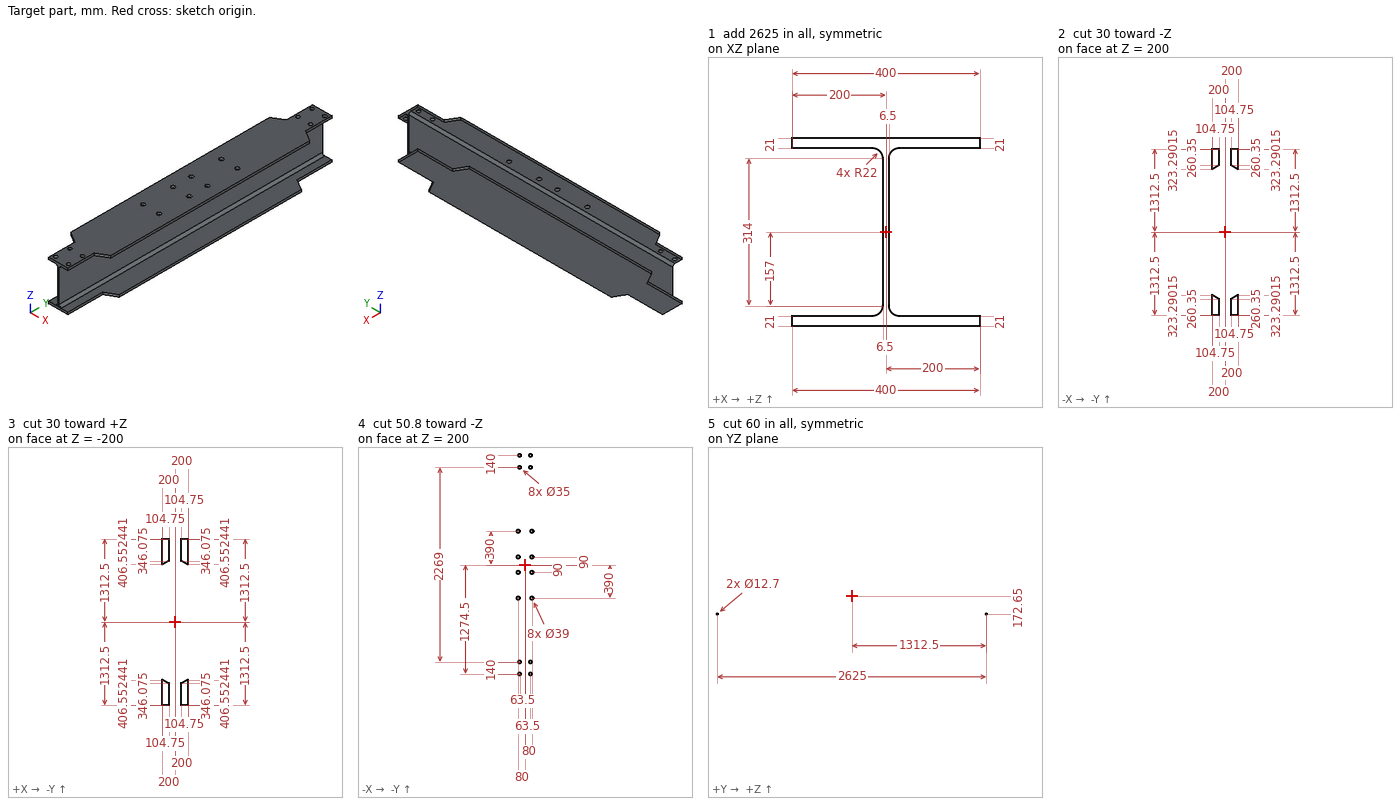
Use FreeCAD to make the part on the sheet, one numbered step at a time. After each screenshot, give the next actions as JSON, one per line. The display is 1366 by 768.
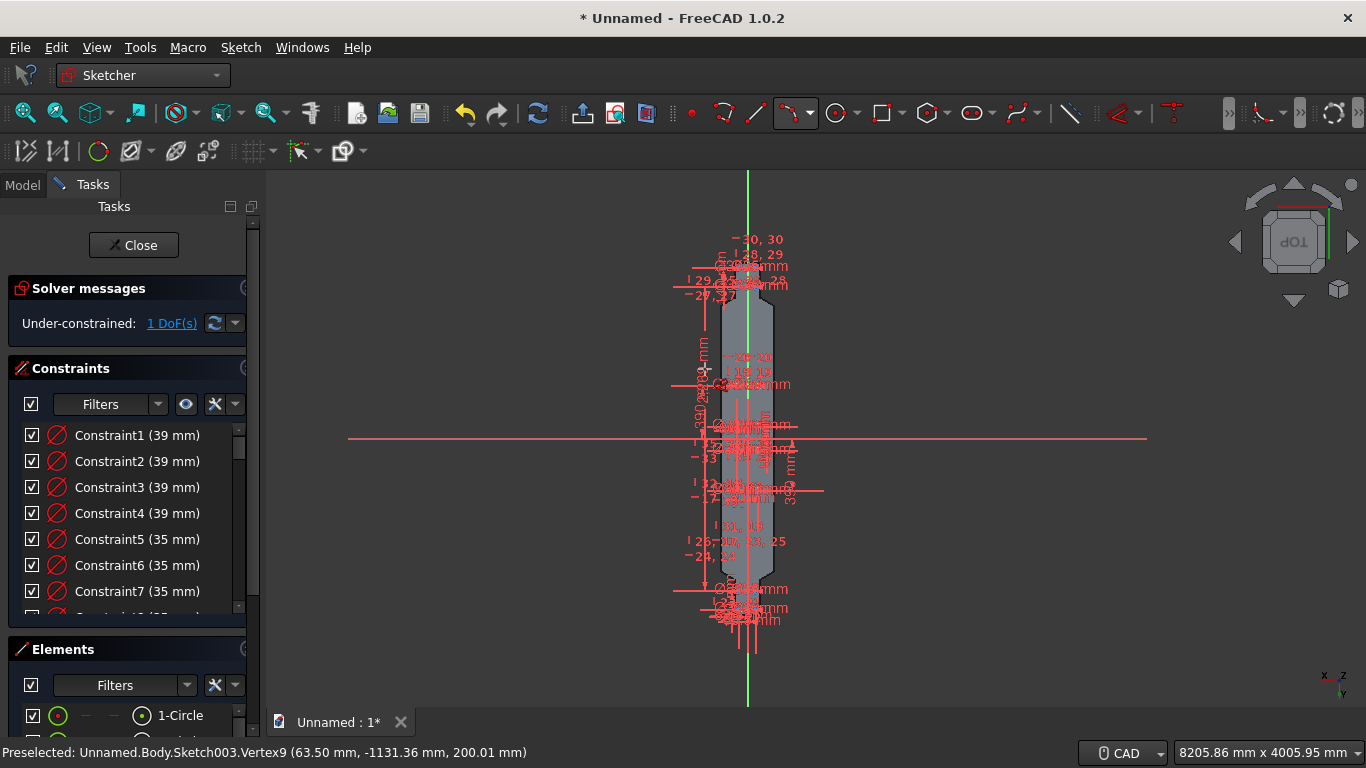
{"action": "left_click", "coordinate": [739, 610]}
{"action": "left_click", "coordinate": [705, 524]}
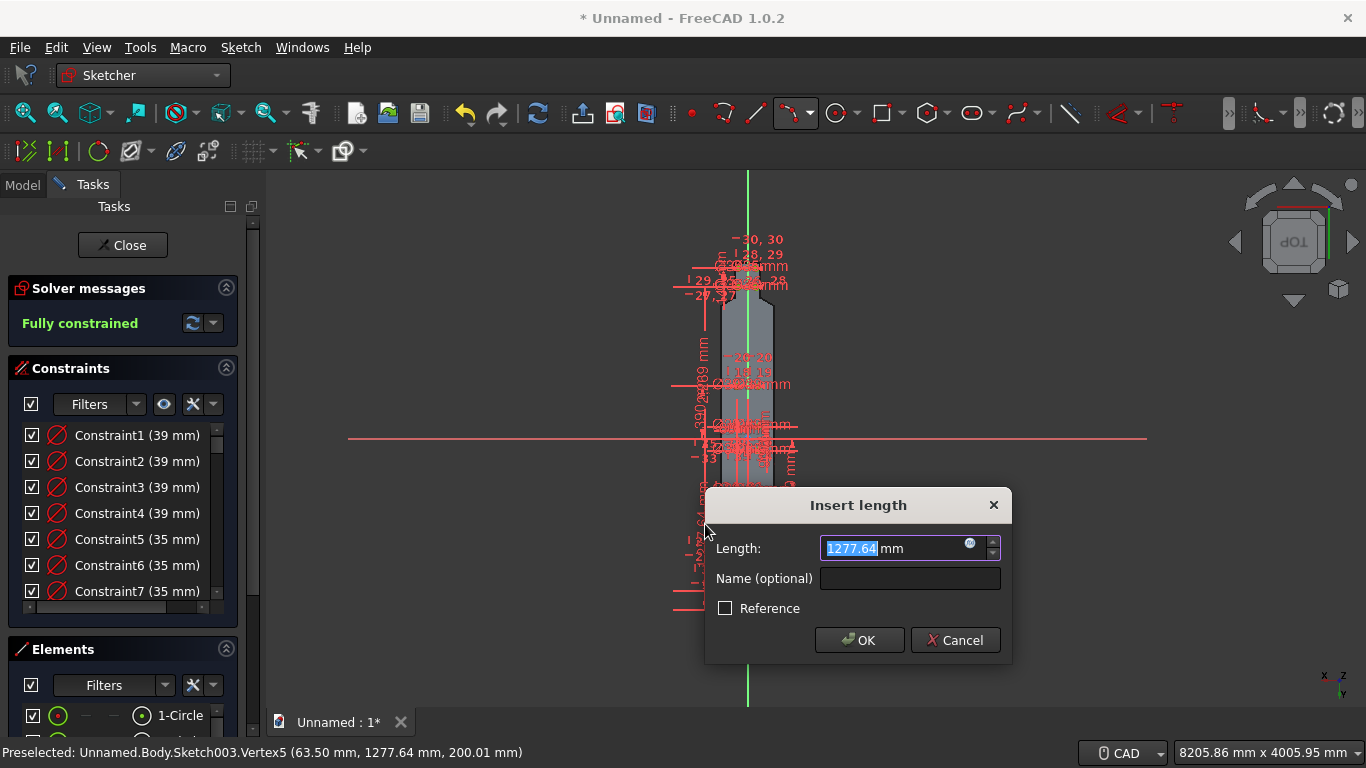
{"action": "type", "text": "1274.5"}
{"action": "key", "text": "Return"}
{"action": "key", "text": "Escape"}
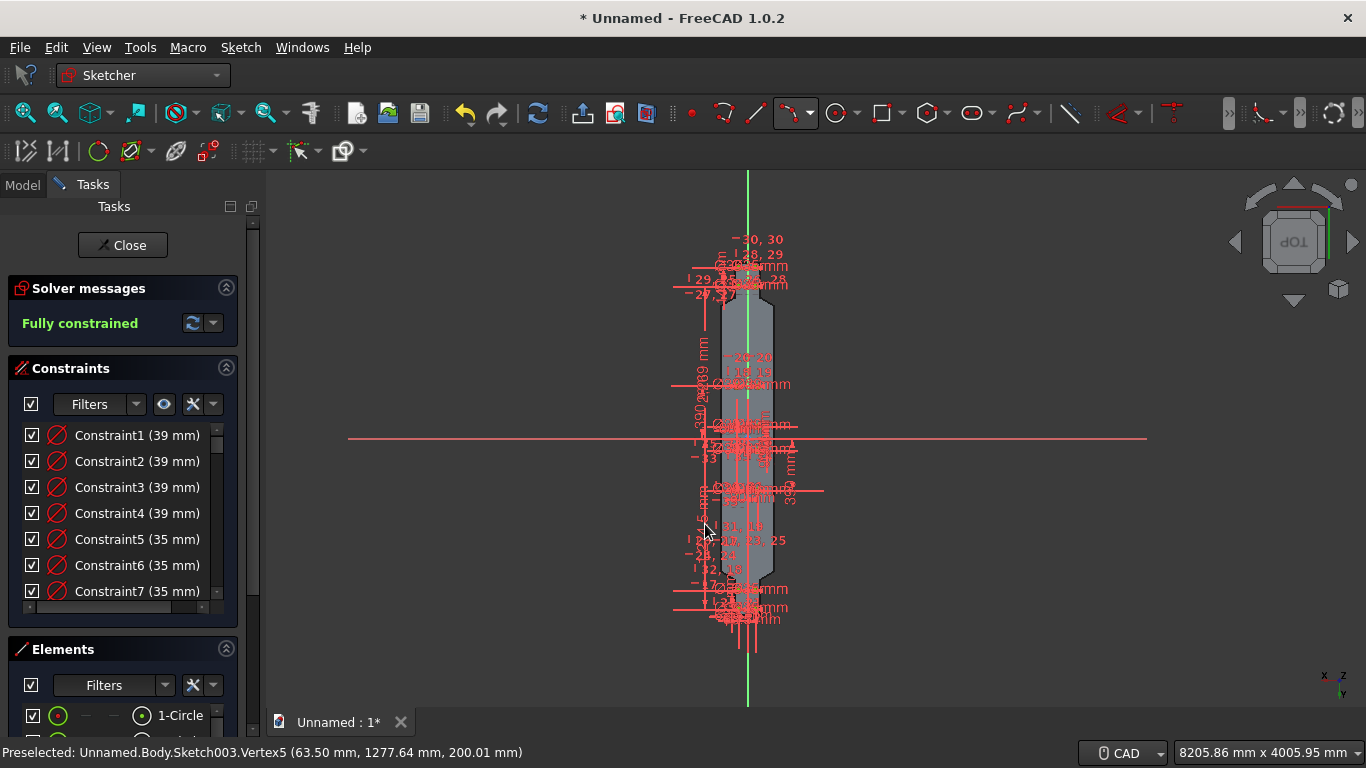
{"action": "left_click", "coordinate": [123, 245]}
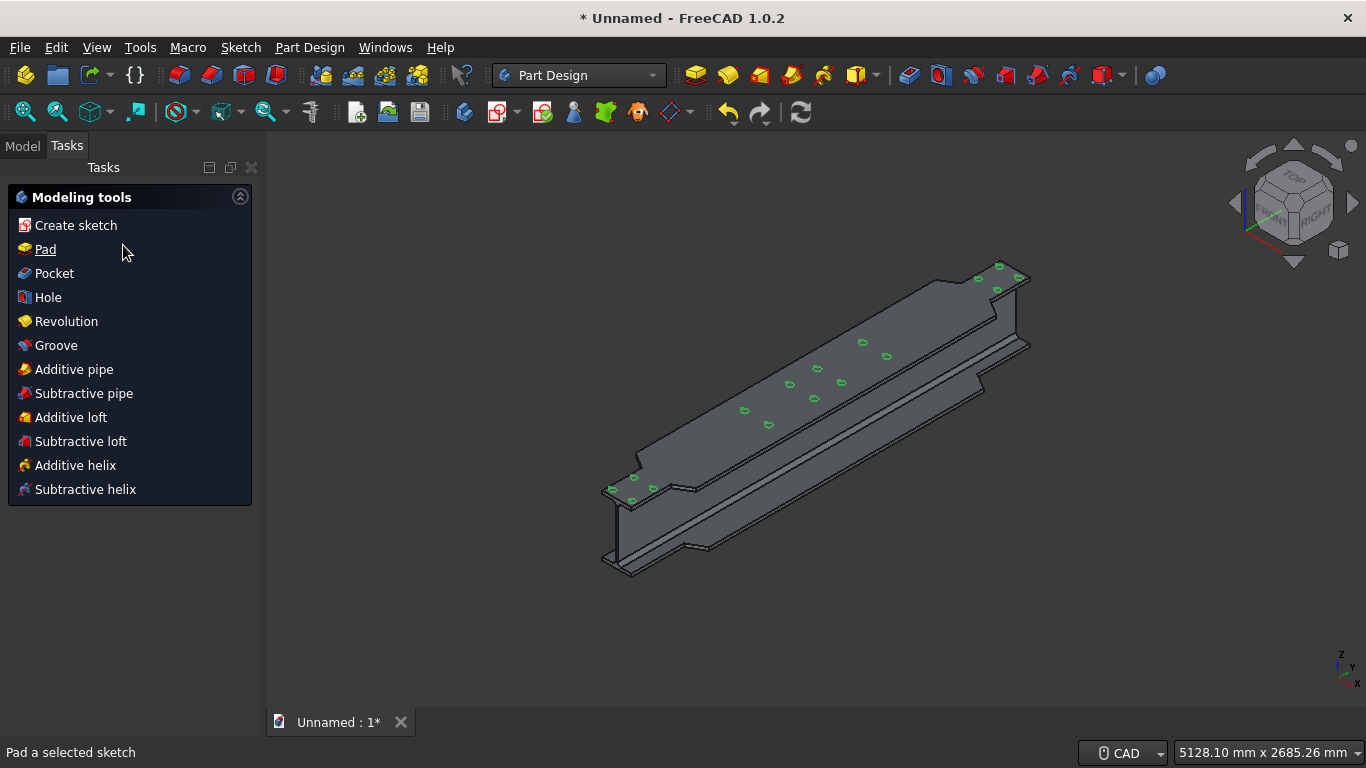
{"action": "left_click", "coordinate": [910, 76]}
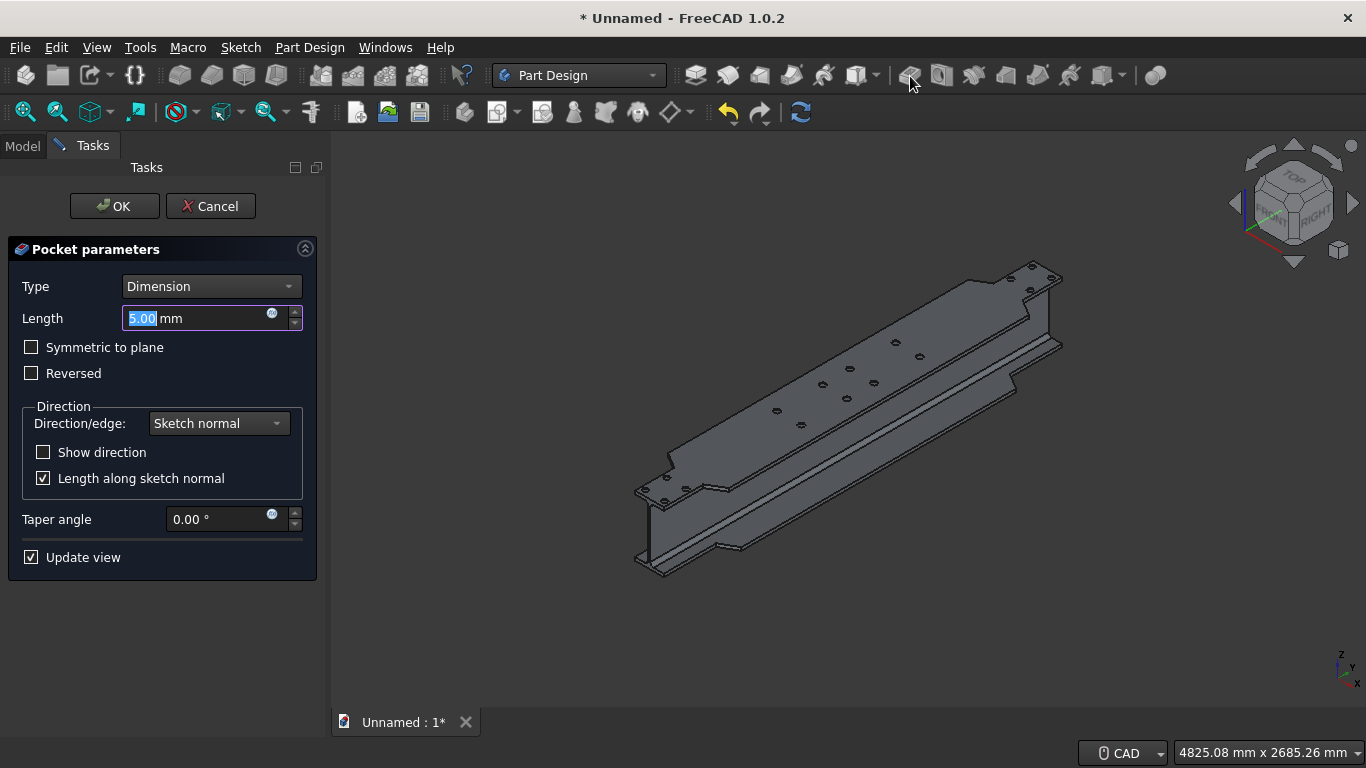
{"action": "type", "text": "50.8"}
{"action": "key", "text": "Tab"}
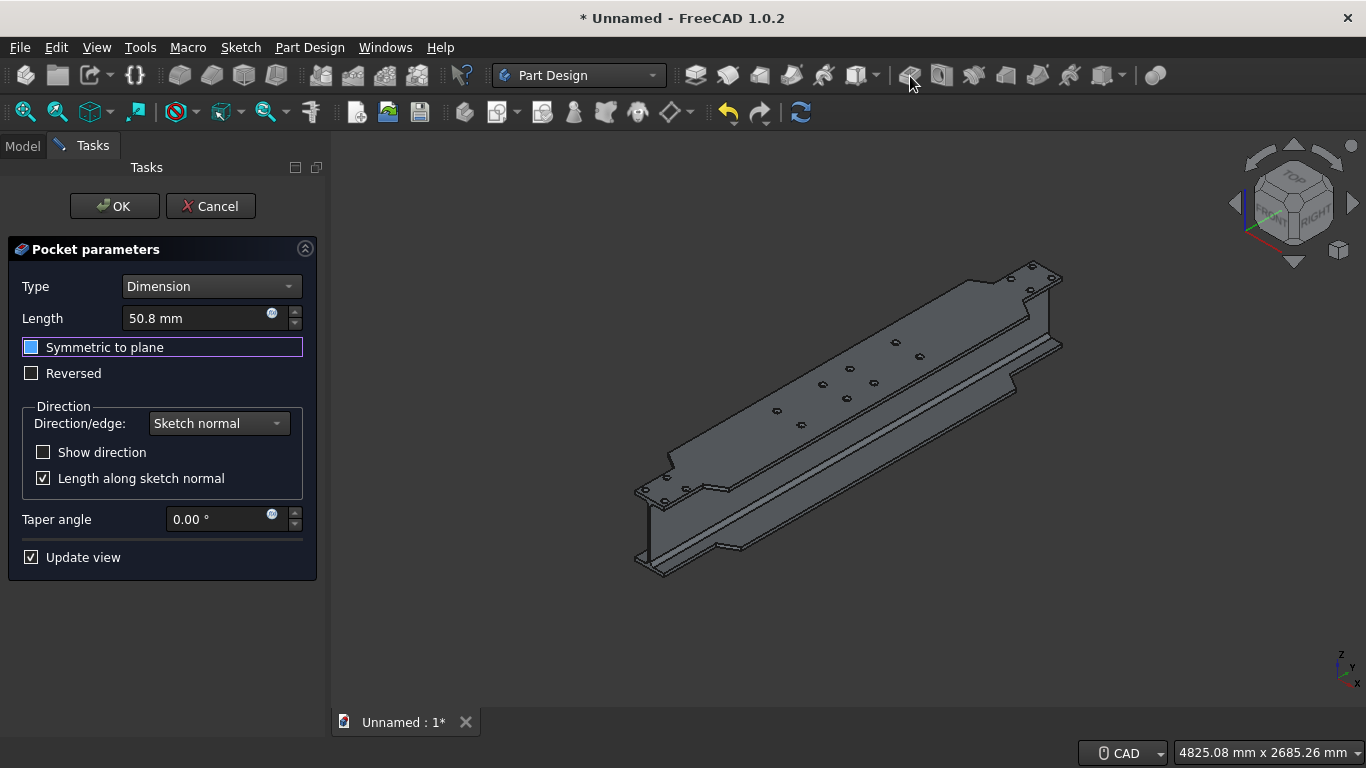
{"action": "left_click", "coordinate": [115, 206]}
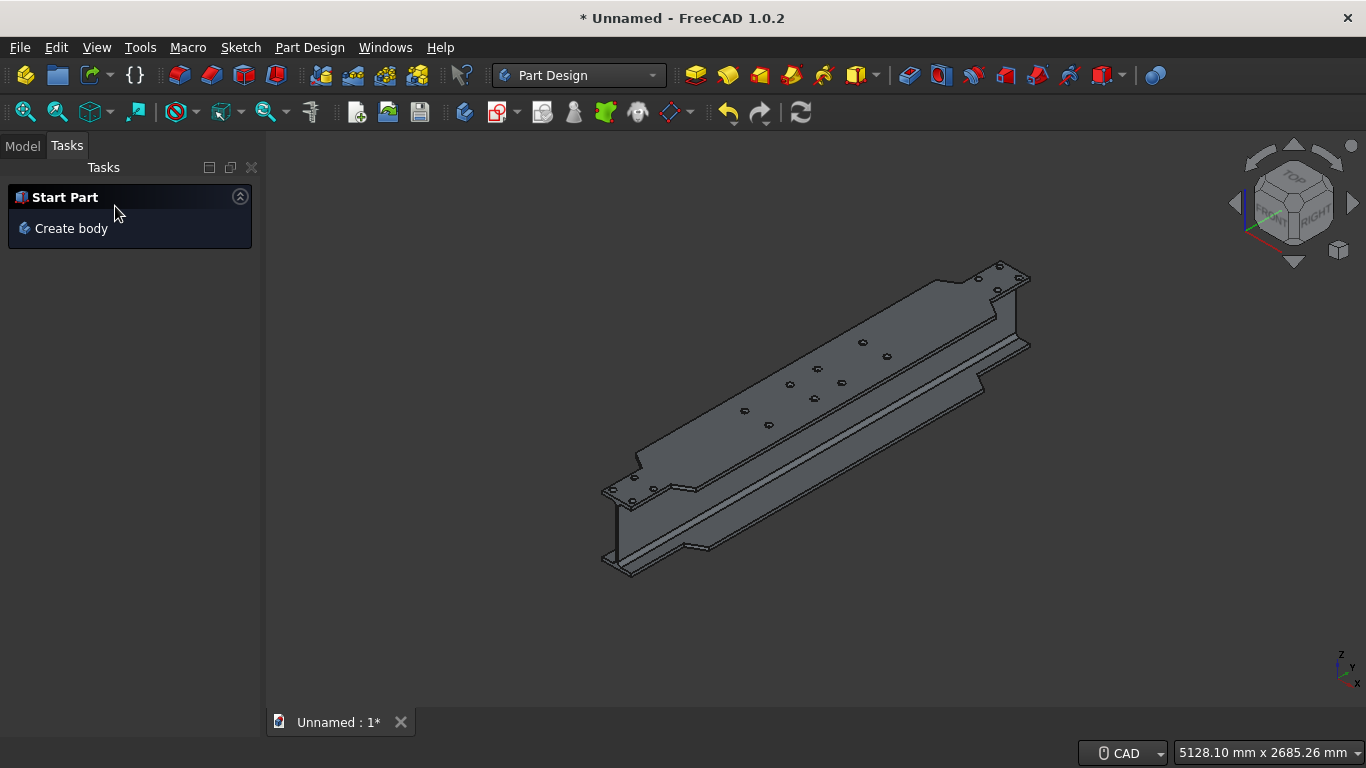
{"action": "left_click", "coordinate": [498, 112]}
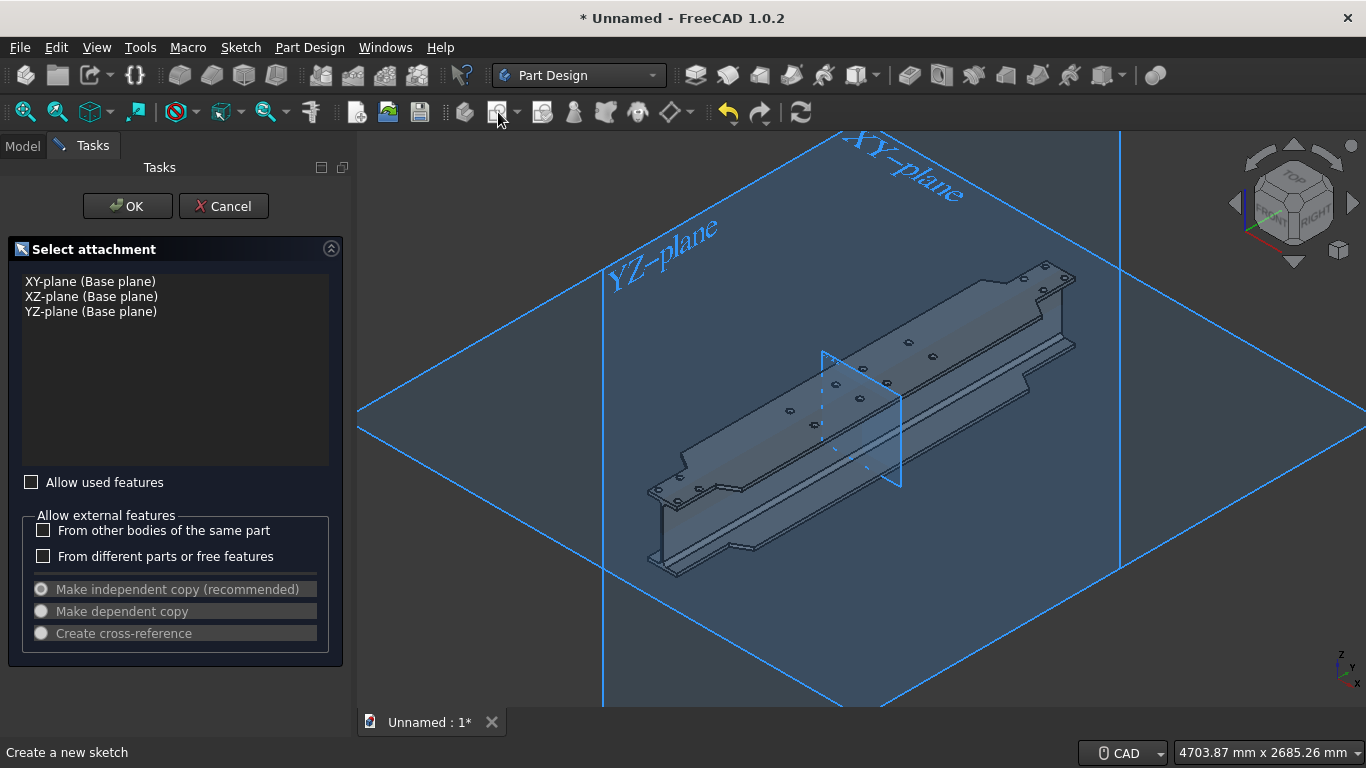
{"action": "left_click", "coordinate": [82, 312]}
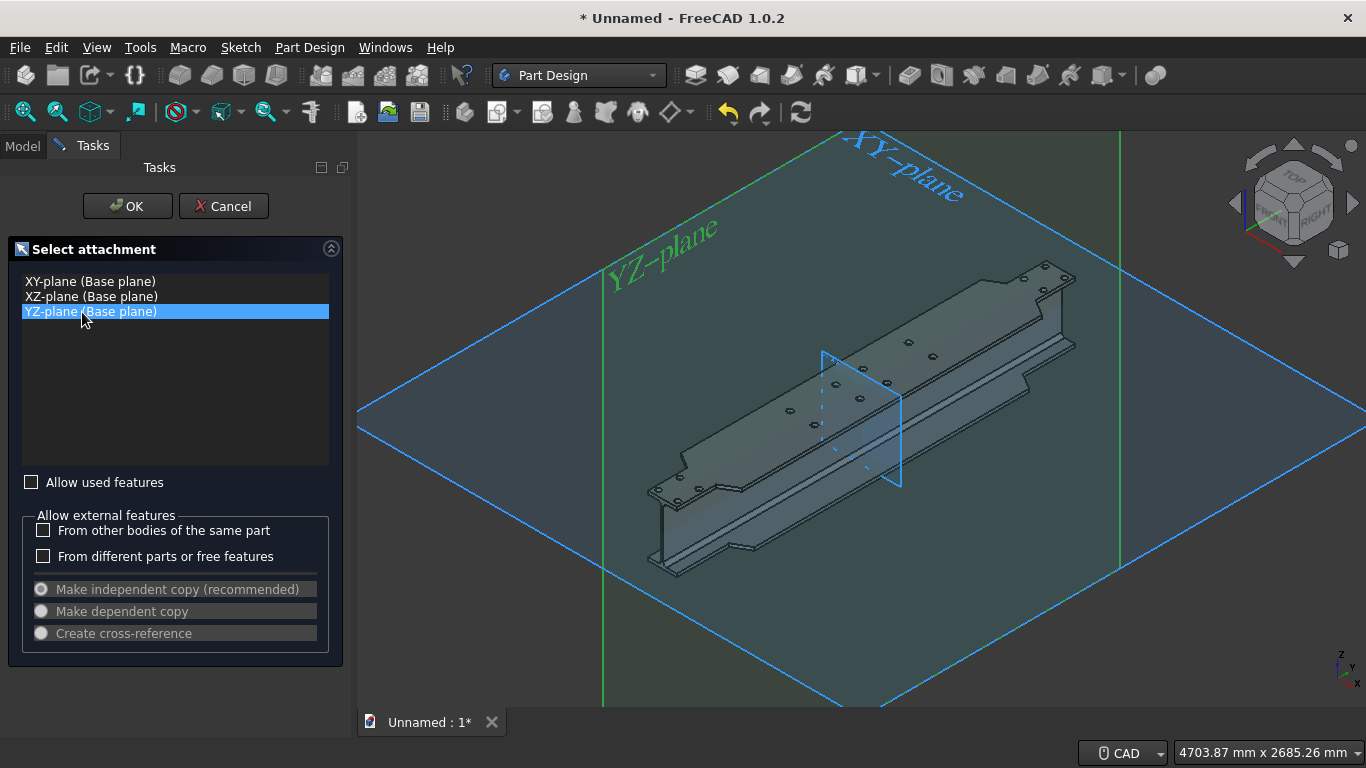
{"action": "left_click", "coordinate": [128, 206]}